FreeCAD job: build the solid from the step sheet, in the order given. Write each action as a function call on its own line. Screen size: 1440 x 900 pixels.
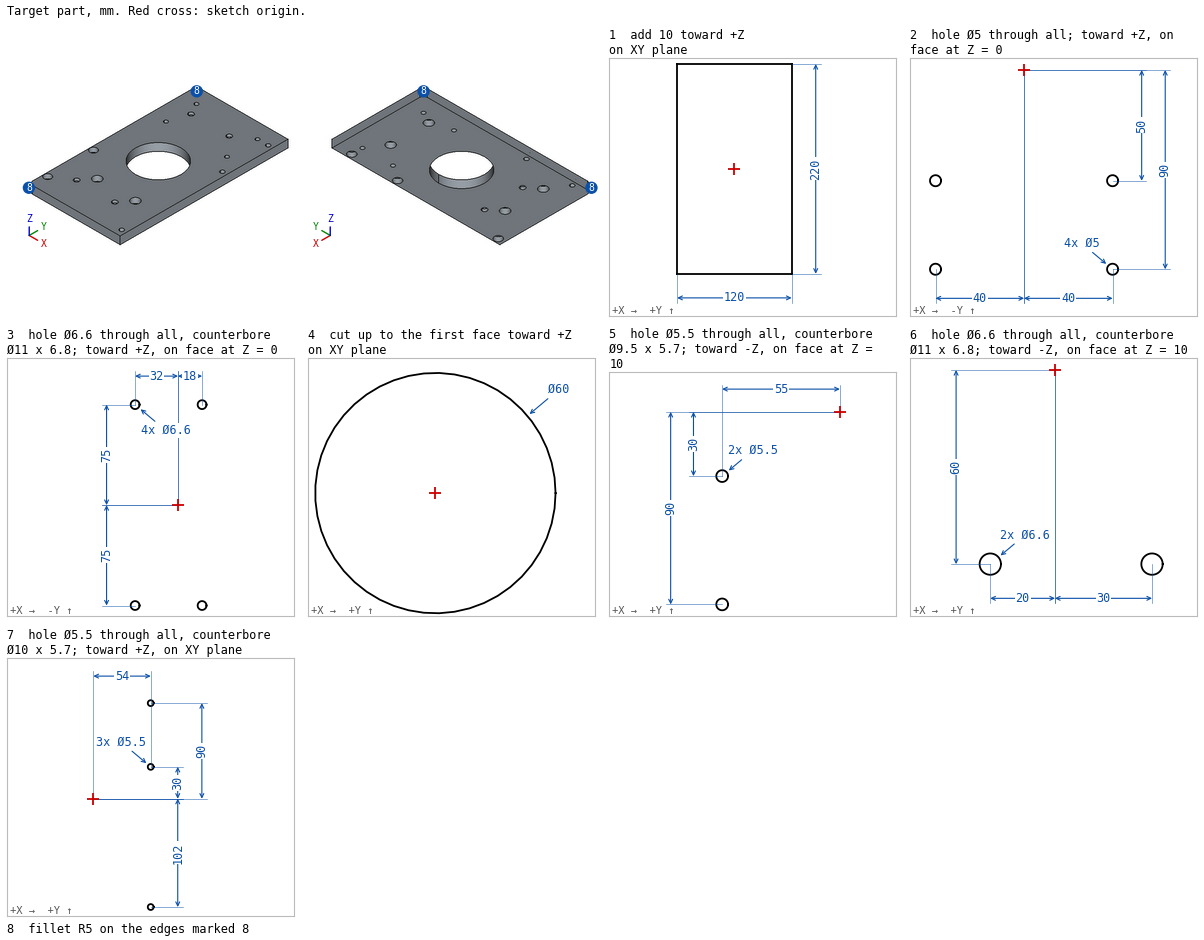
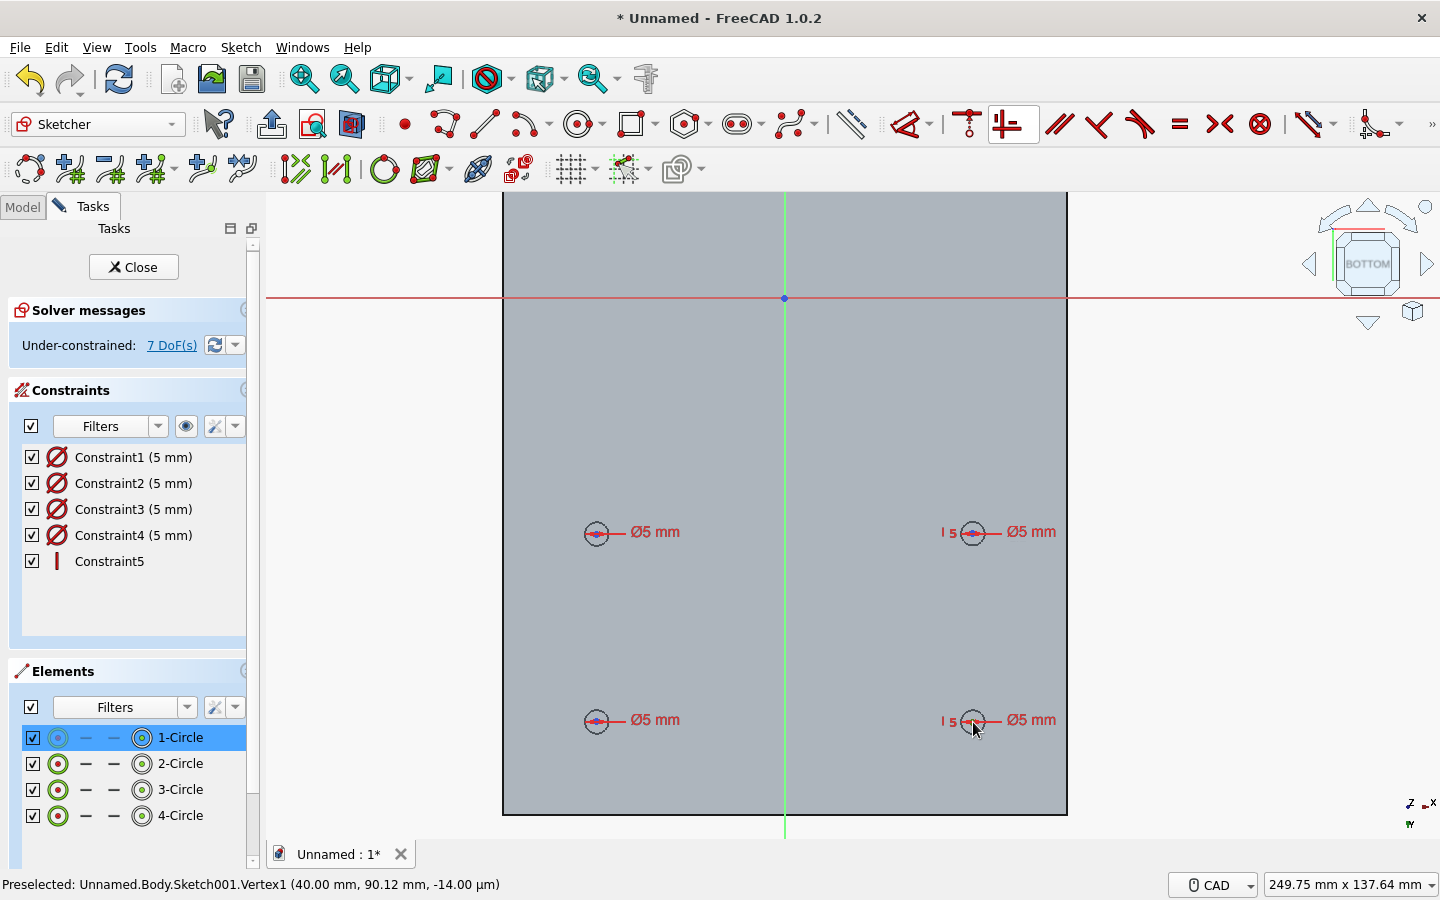
click(597, 722)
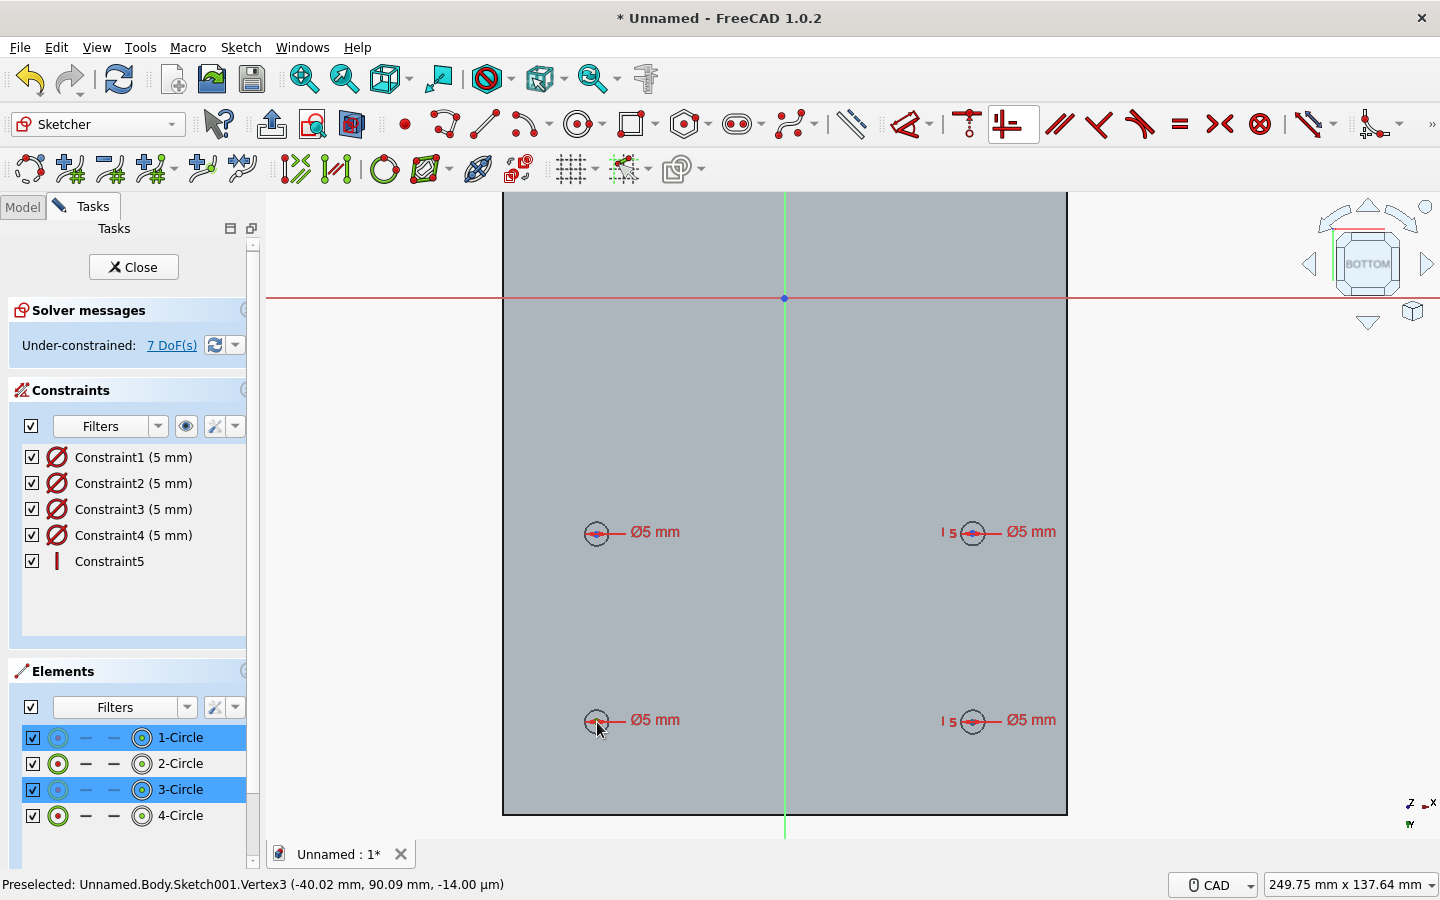
key(h)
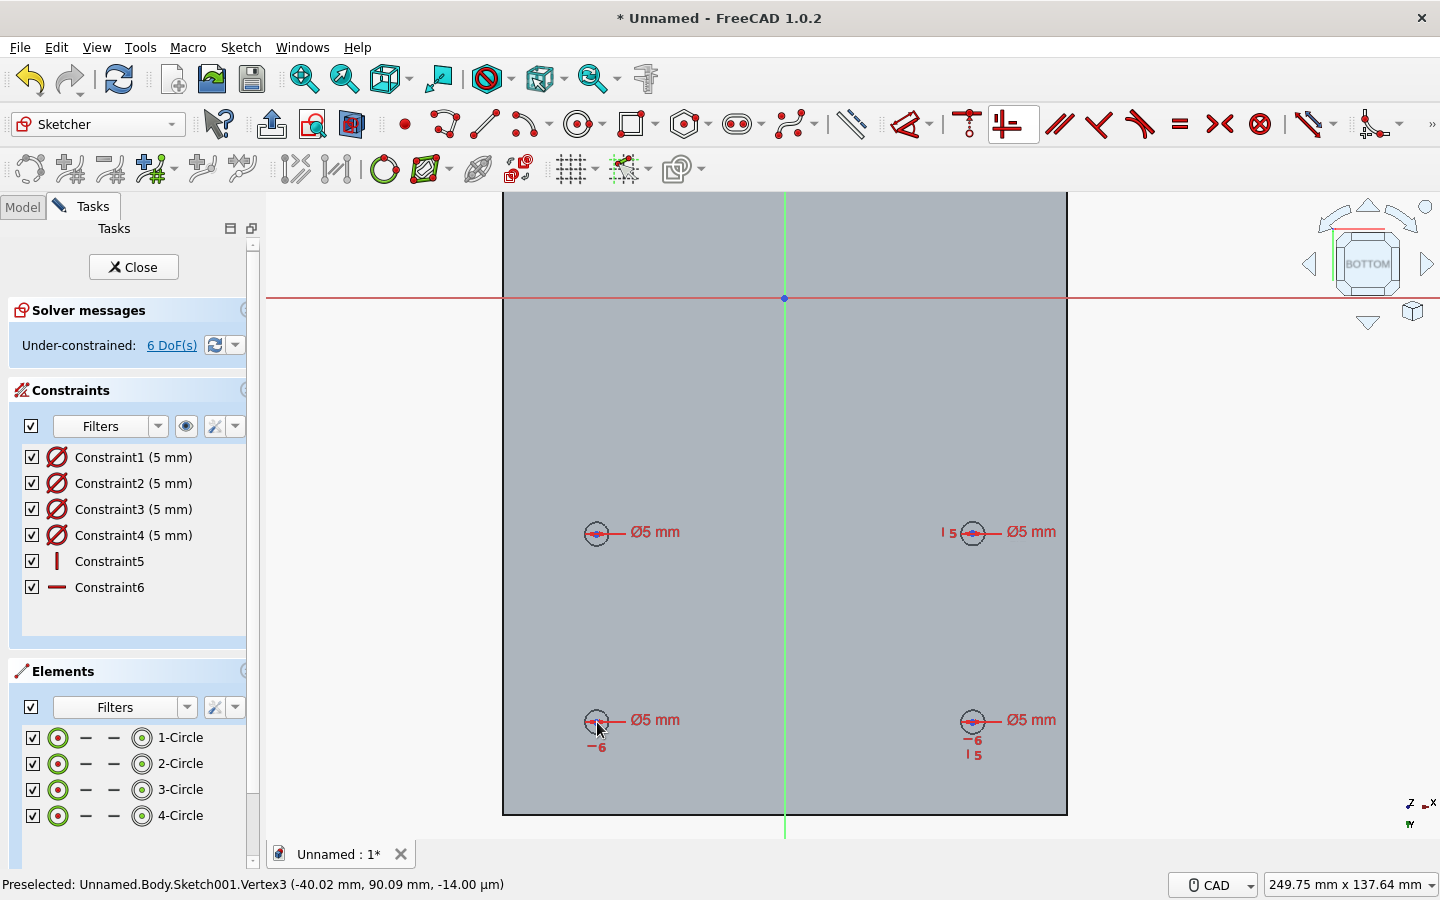
click(597, 722)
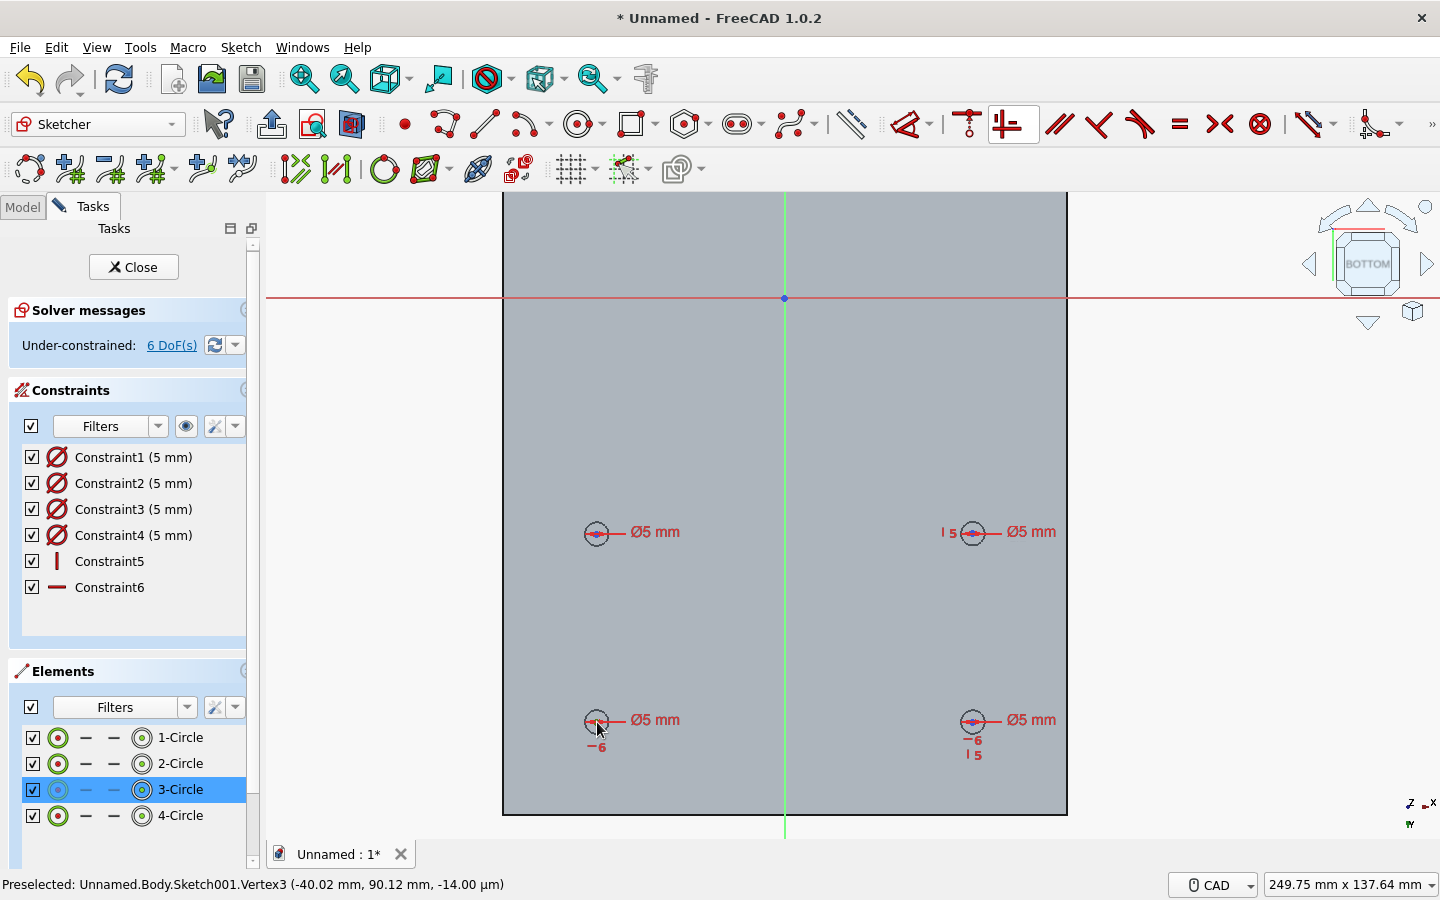
click(597, 534)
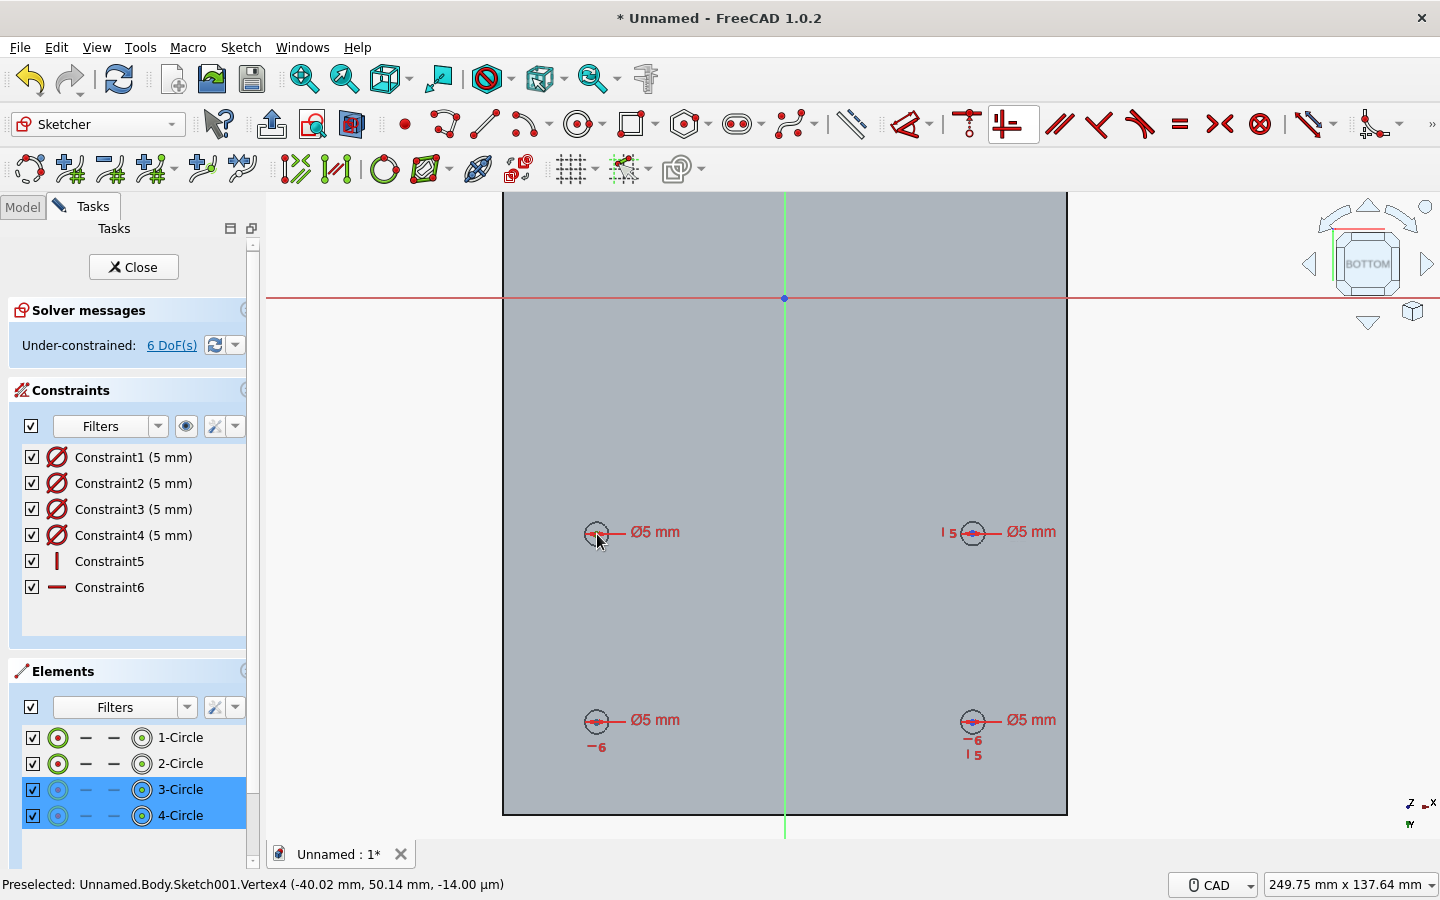
key(v)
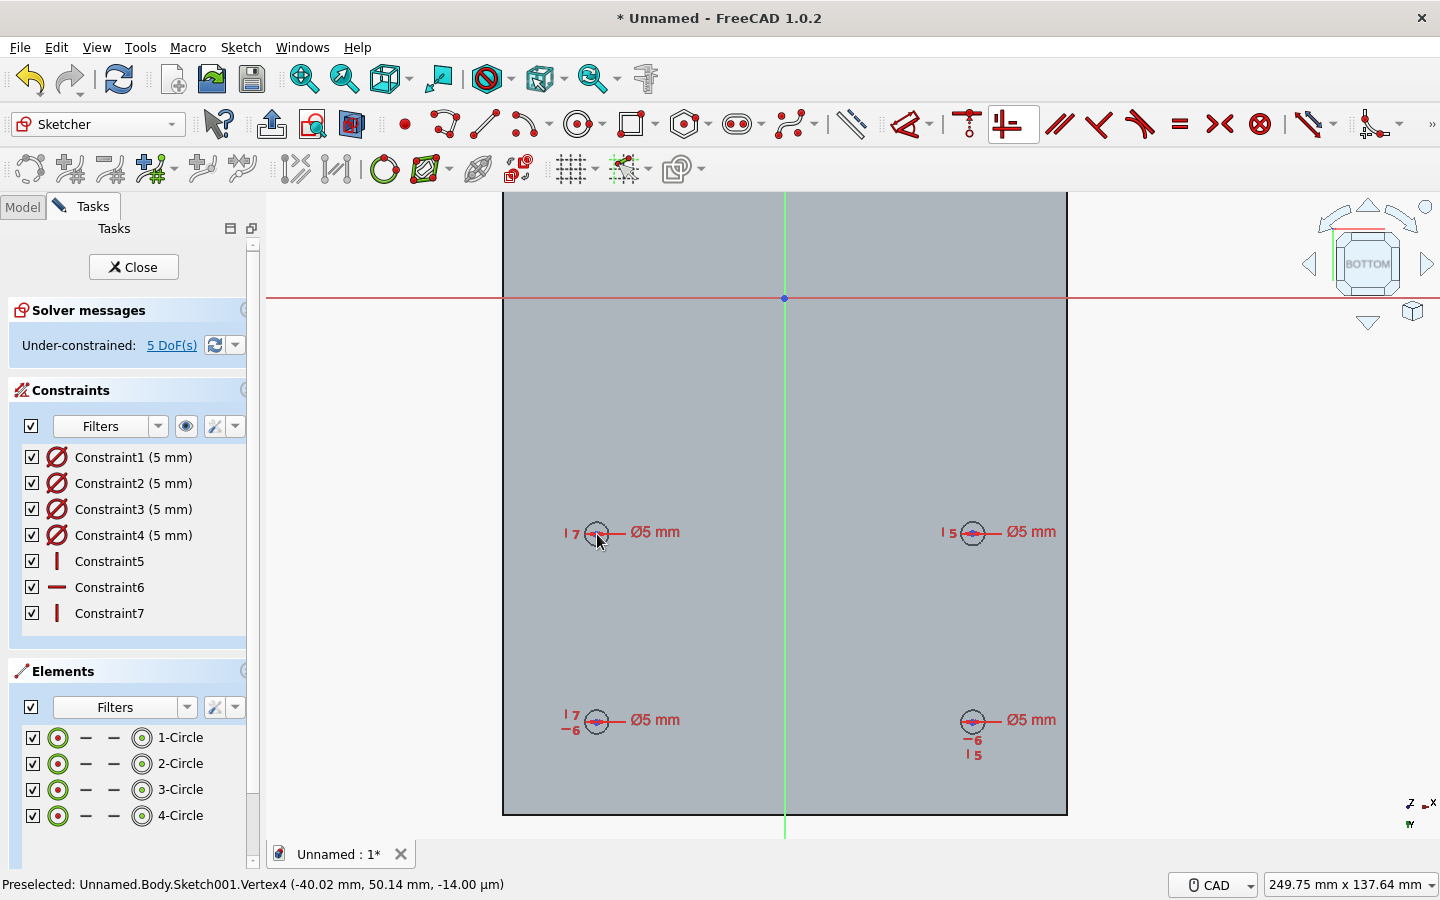
click(973, 534)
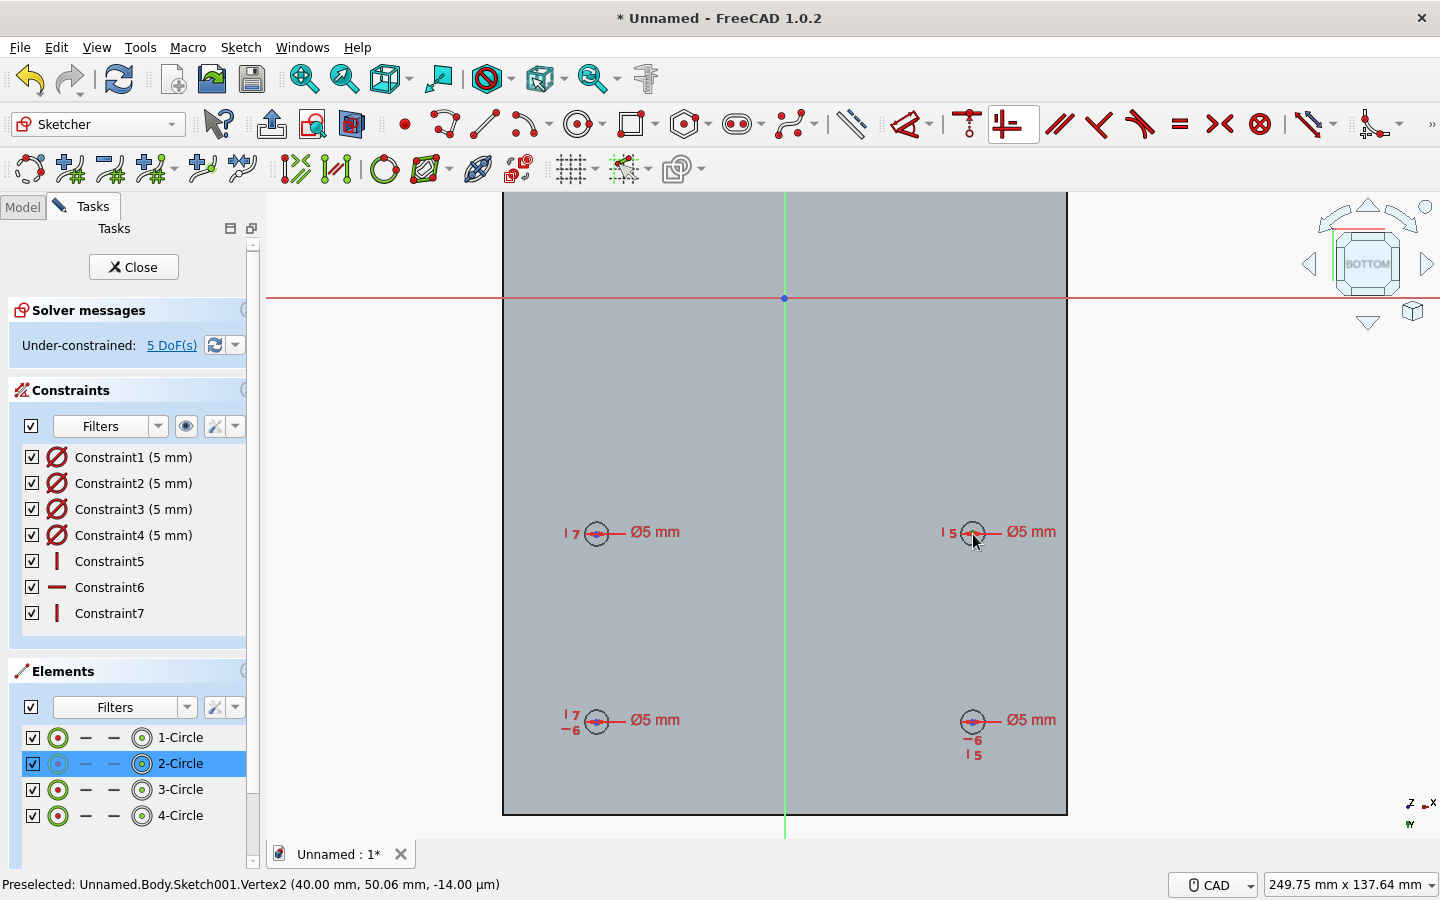
click(597, 534)